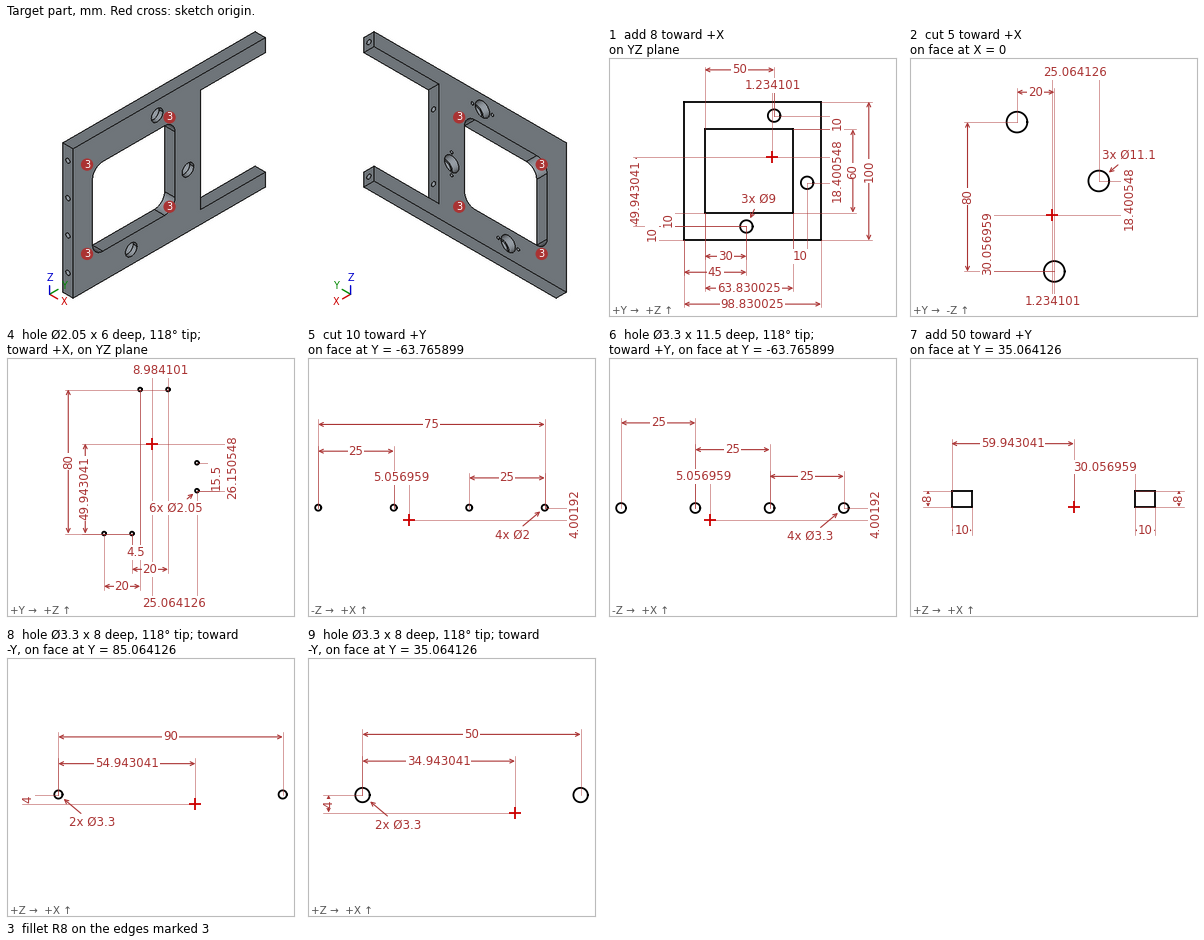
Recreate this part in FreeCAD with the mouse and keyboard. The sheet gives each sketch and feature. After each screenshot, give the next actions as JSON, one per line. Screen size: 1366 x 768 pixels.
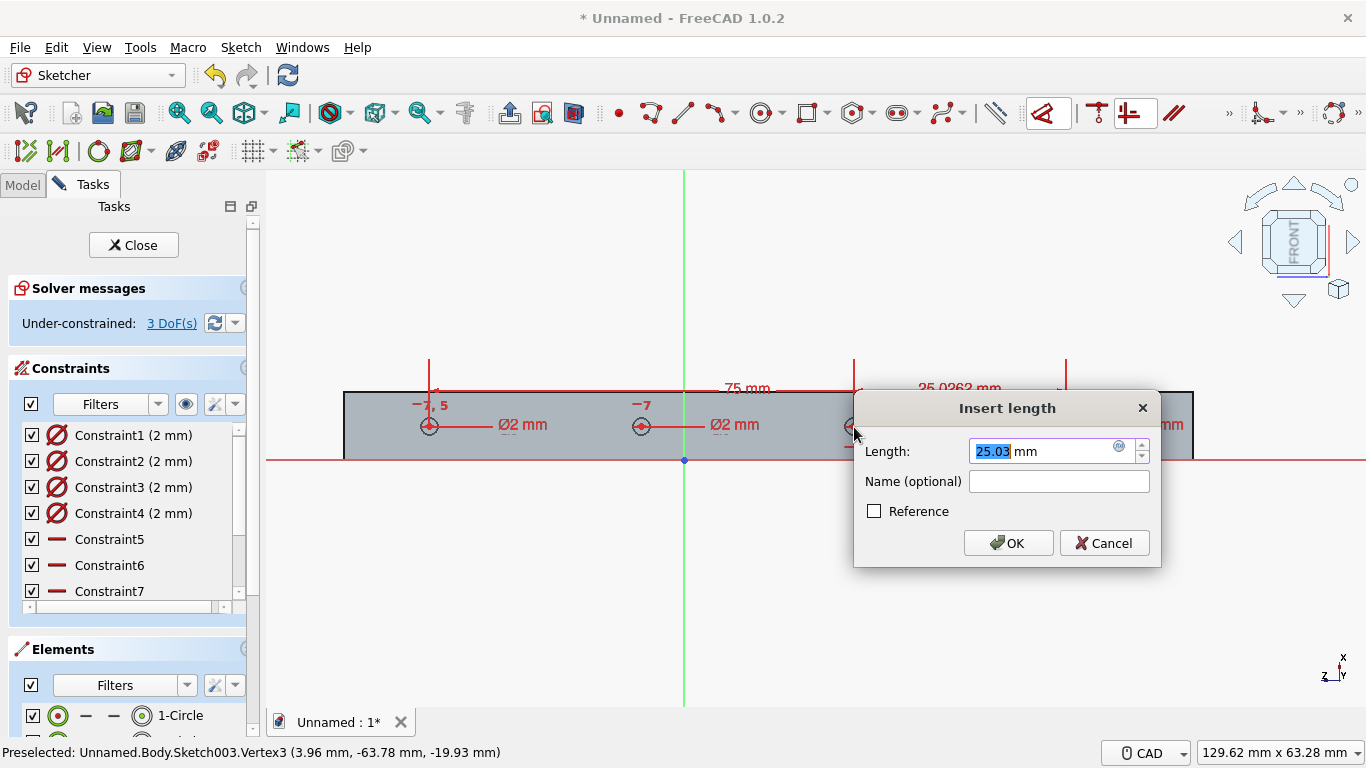
{"action": "type", "text": "25"}
{"action": "key", "text": "Return"}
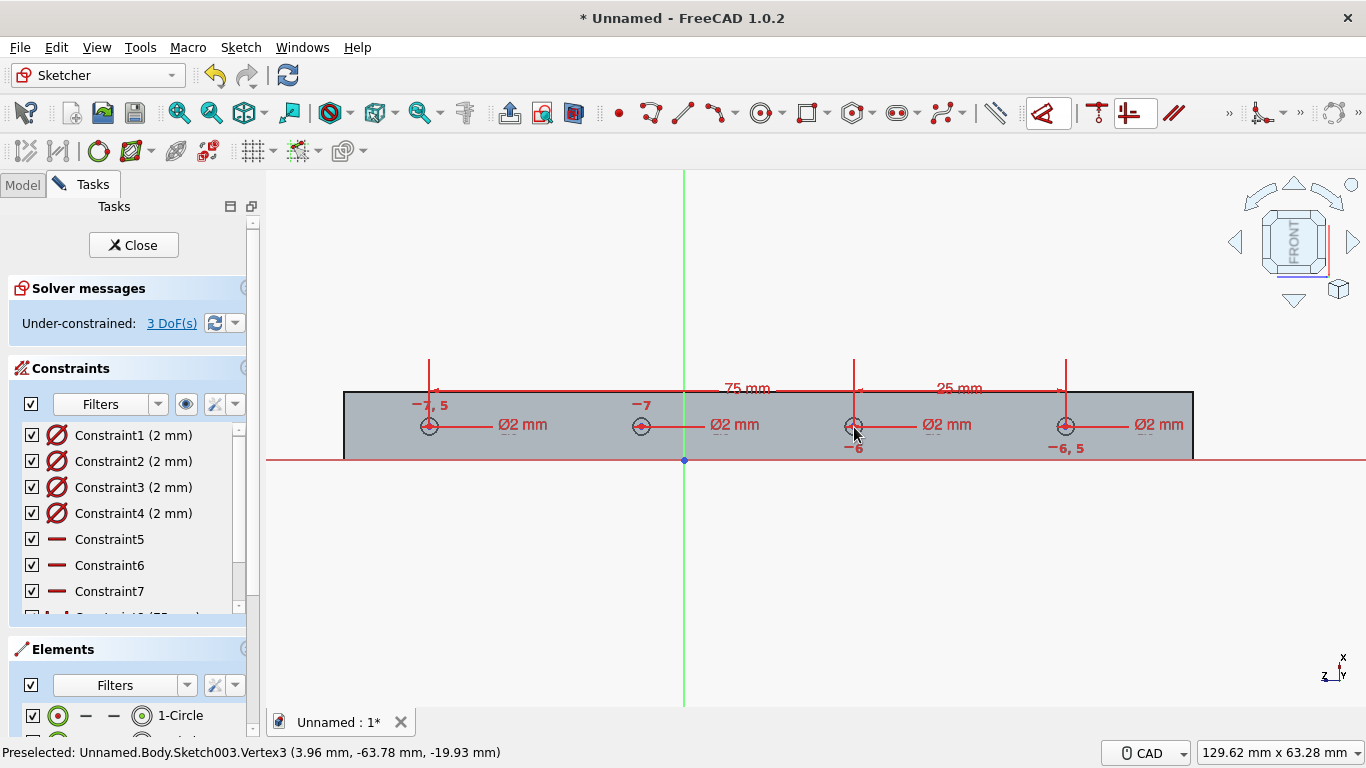
{"action": "left_click", "coordinate": [429, 427]}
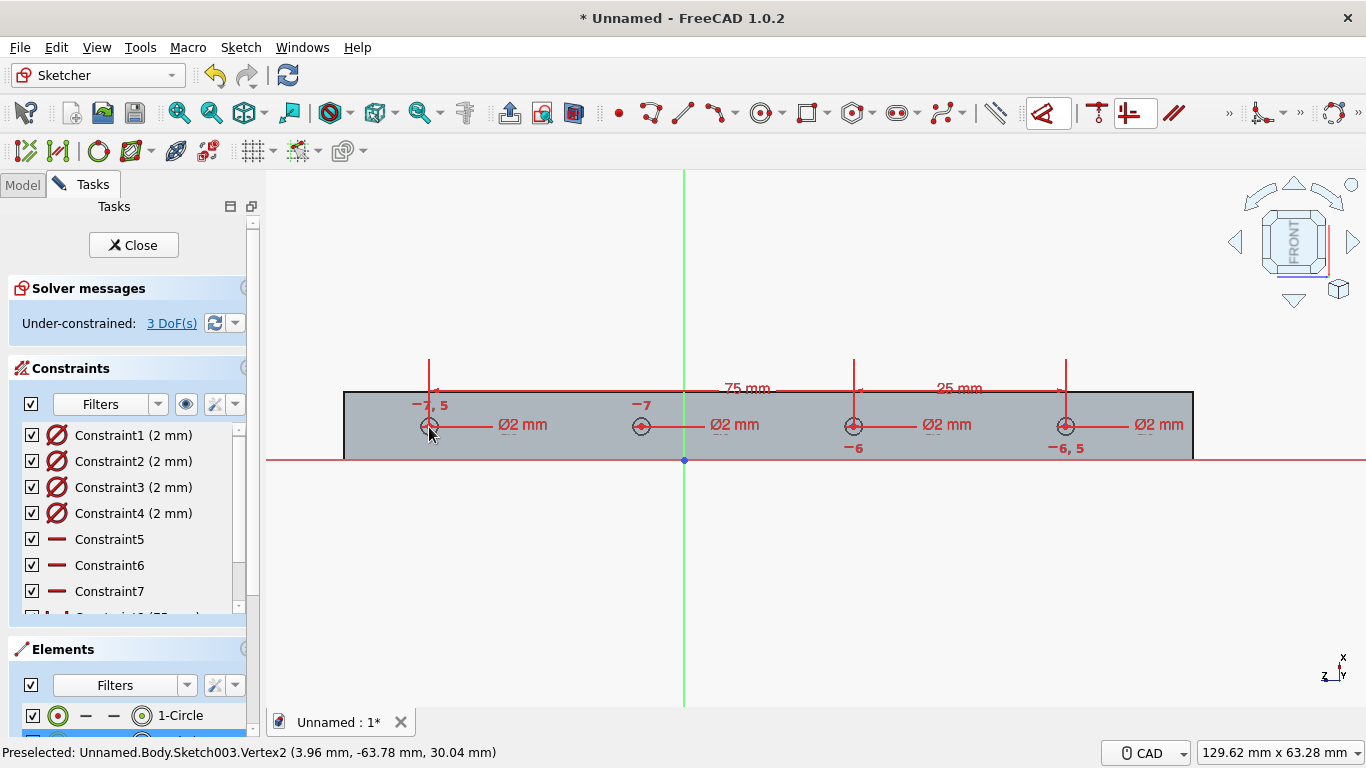
{"action": "left_click", "coordinate": [641, 427]}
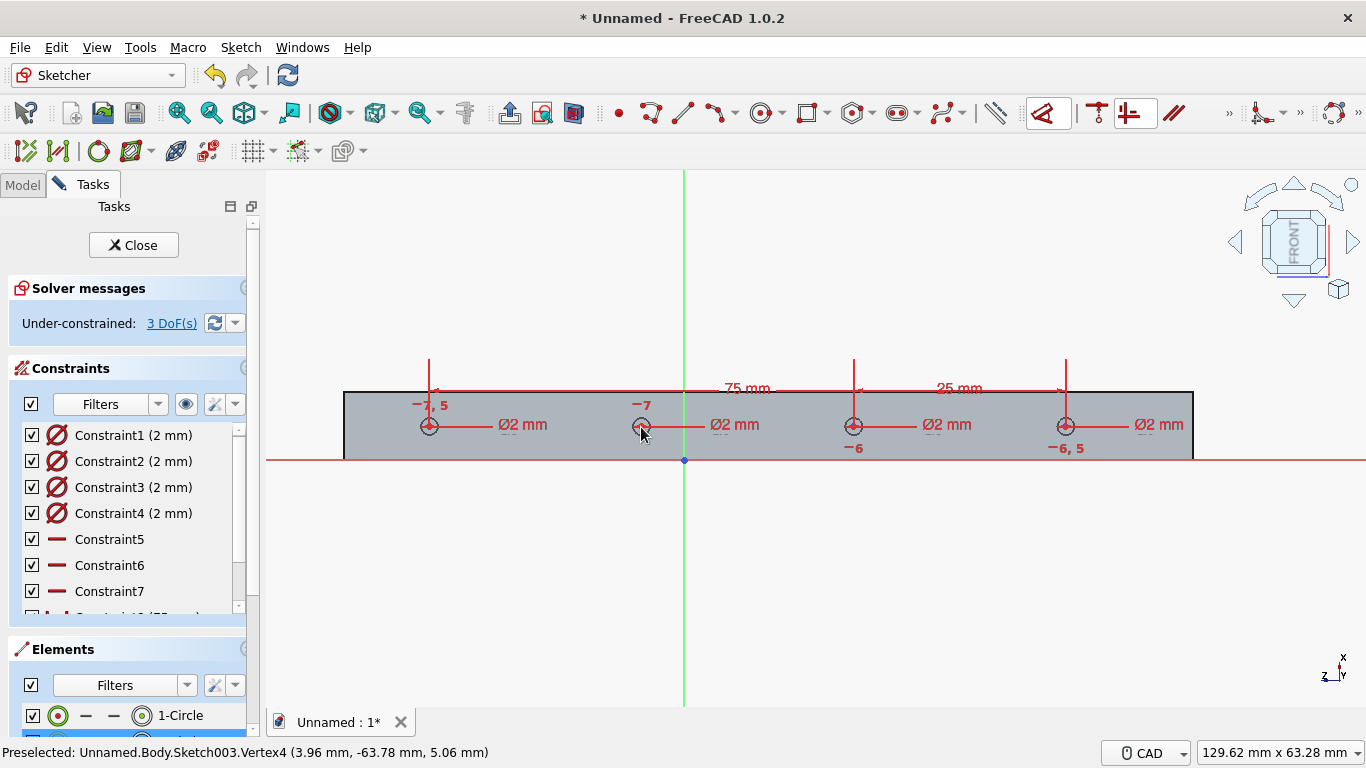
{"action": "left_click", "coordinate": [1066, 114]}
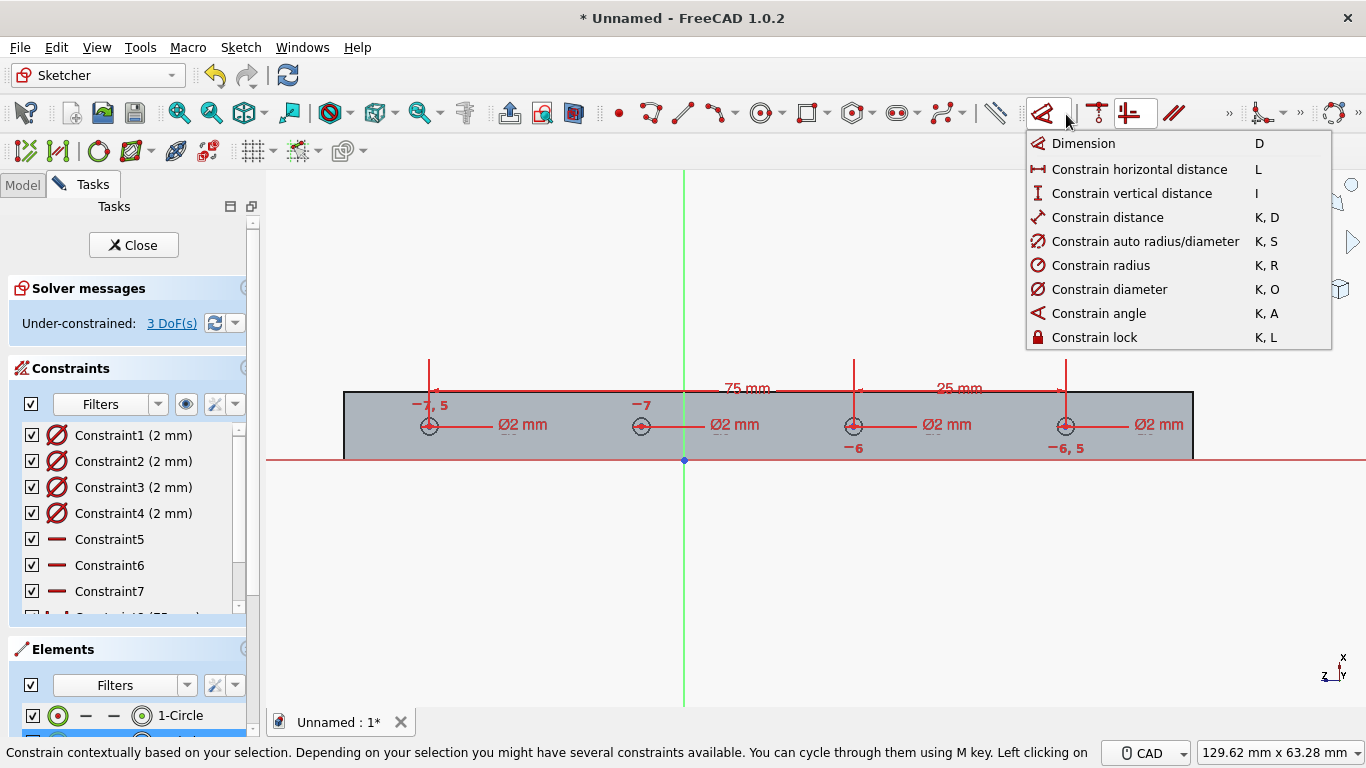
{"action": "left_click", "coordinate": [1179, 169]}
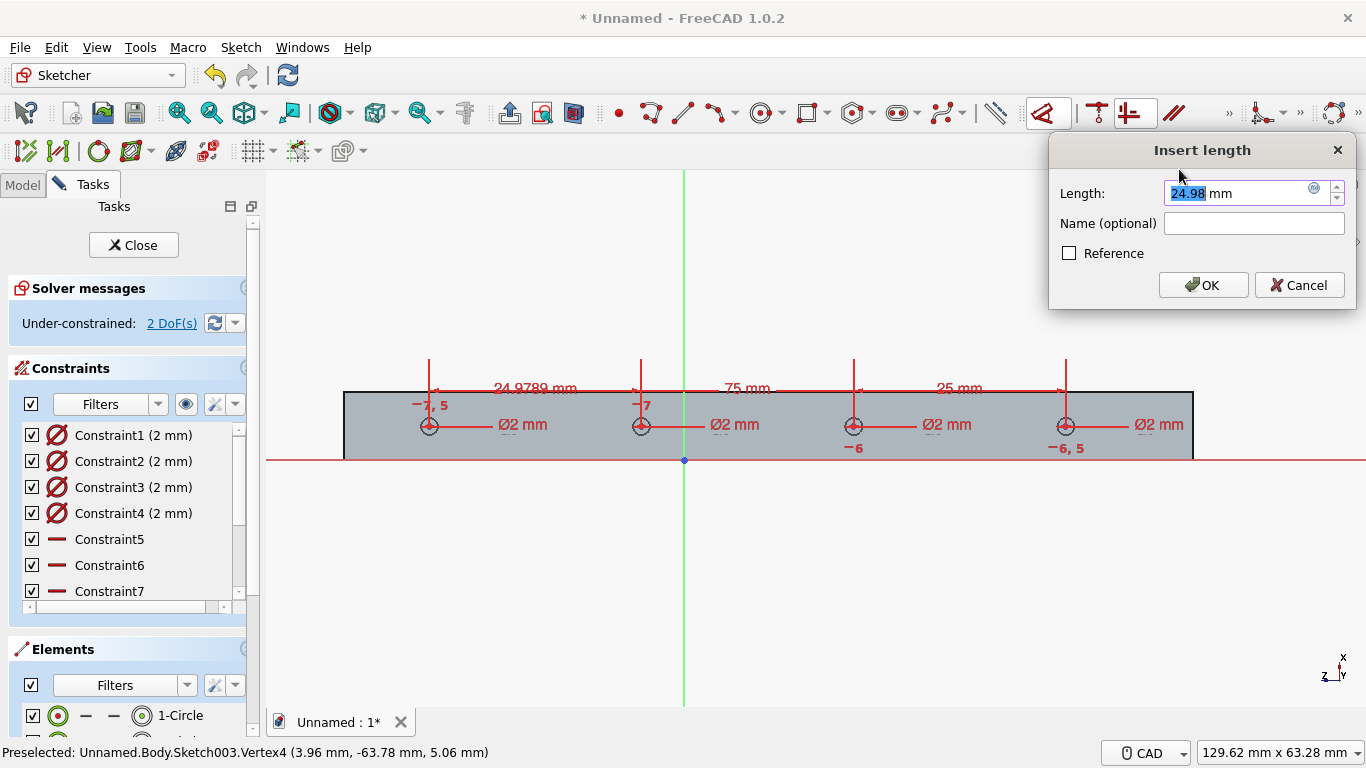
{"action": "type", "text": "25"}
{"action": "key", "text": "Return"}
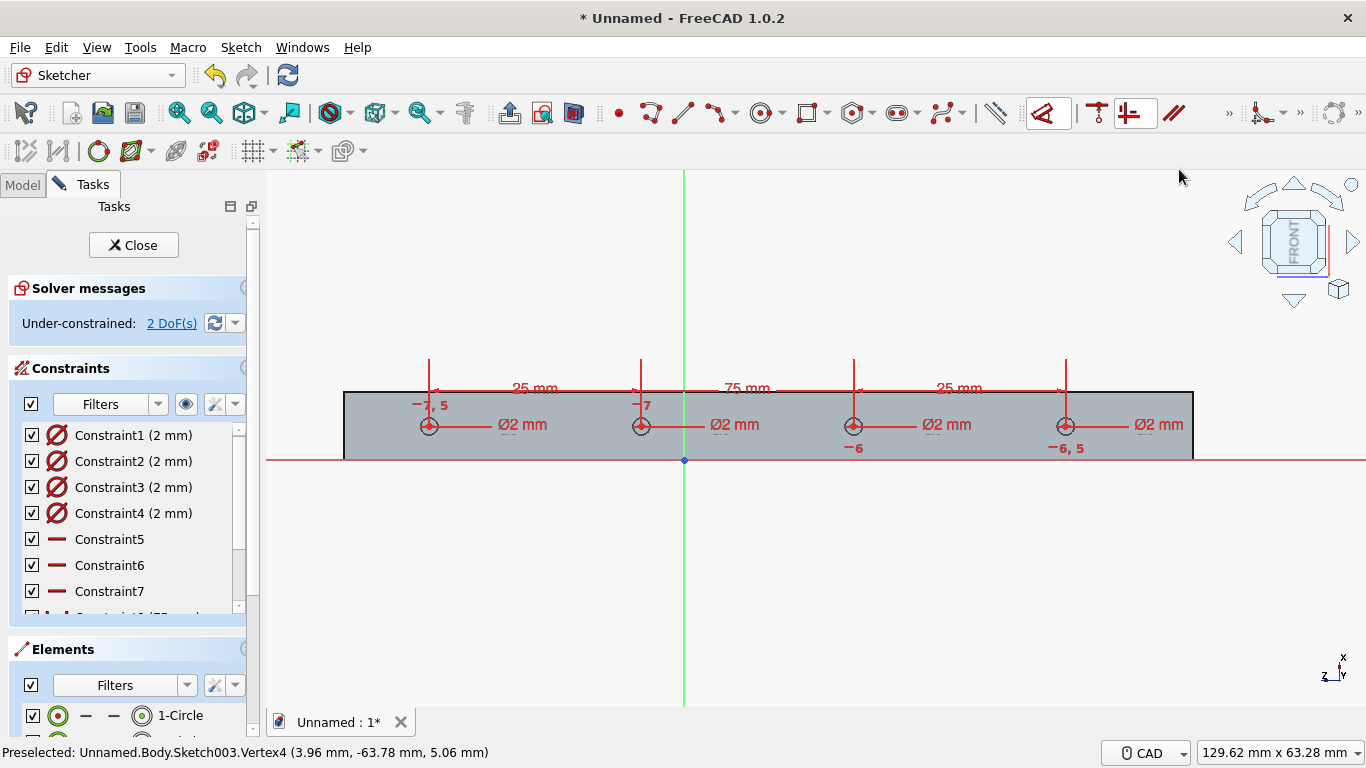
{"action": "left_click", "coordinate": [1066, 427]}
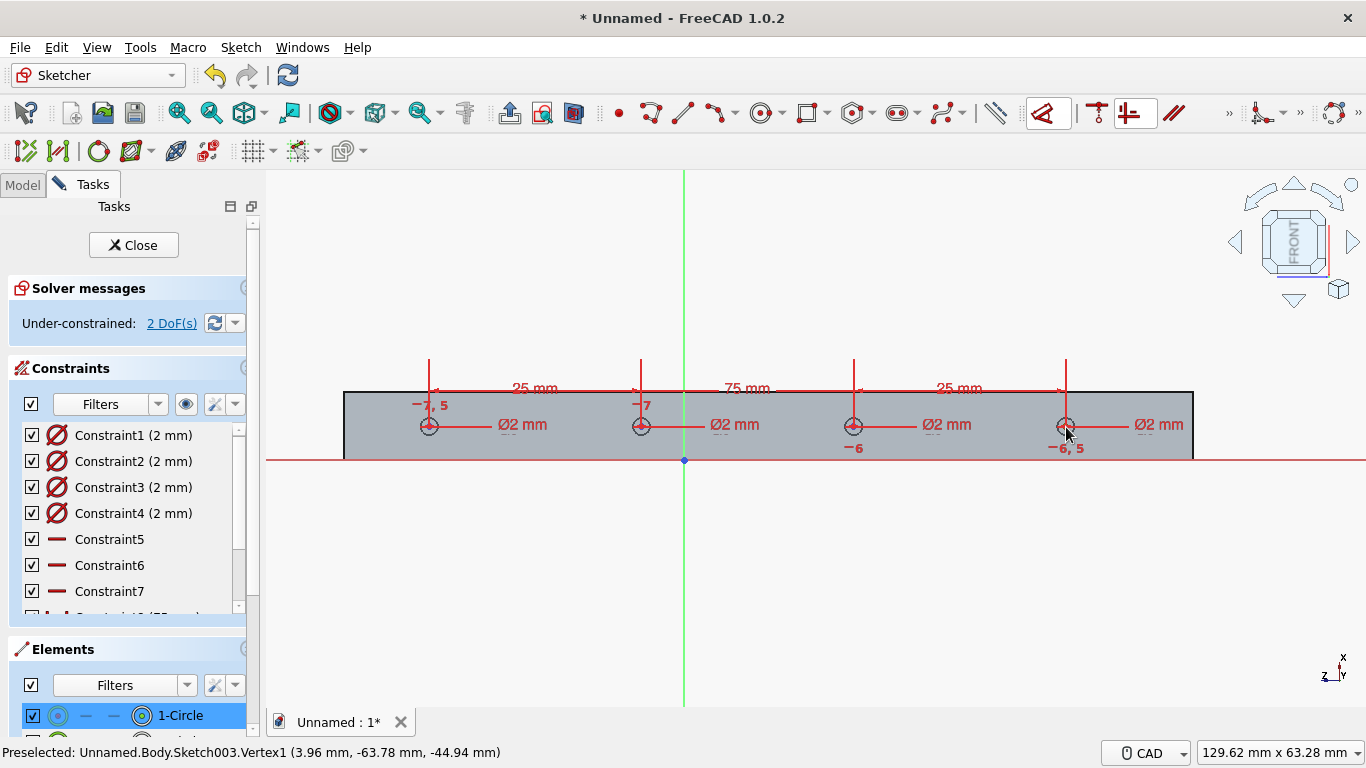
{"action": "left_click", "coordinate": [1066, 114]}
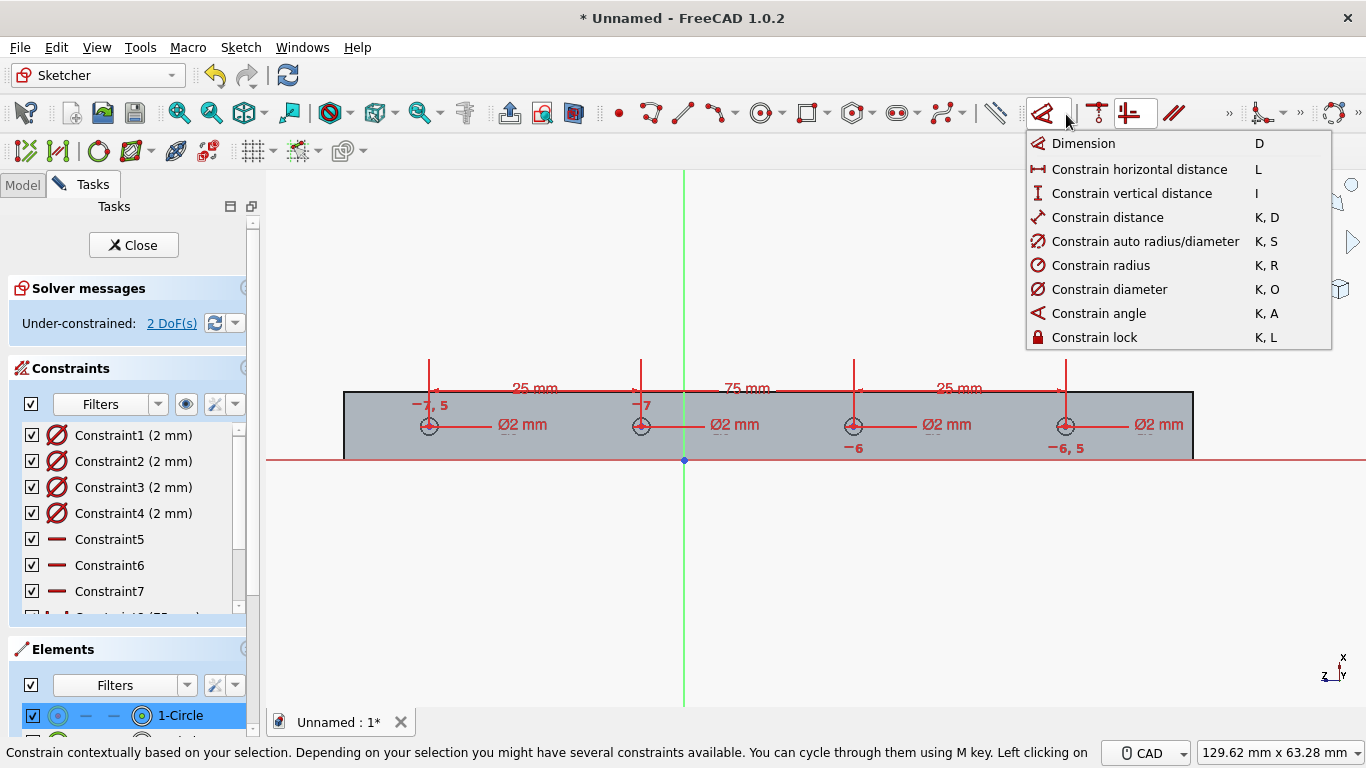
{"action": "left_click", "coordinate": [1179, 193]}